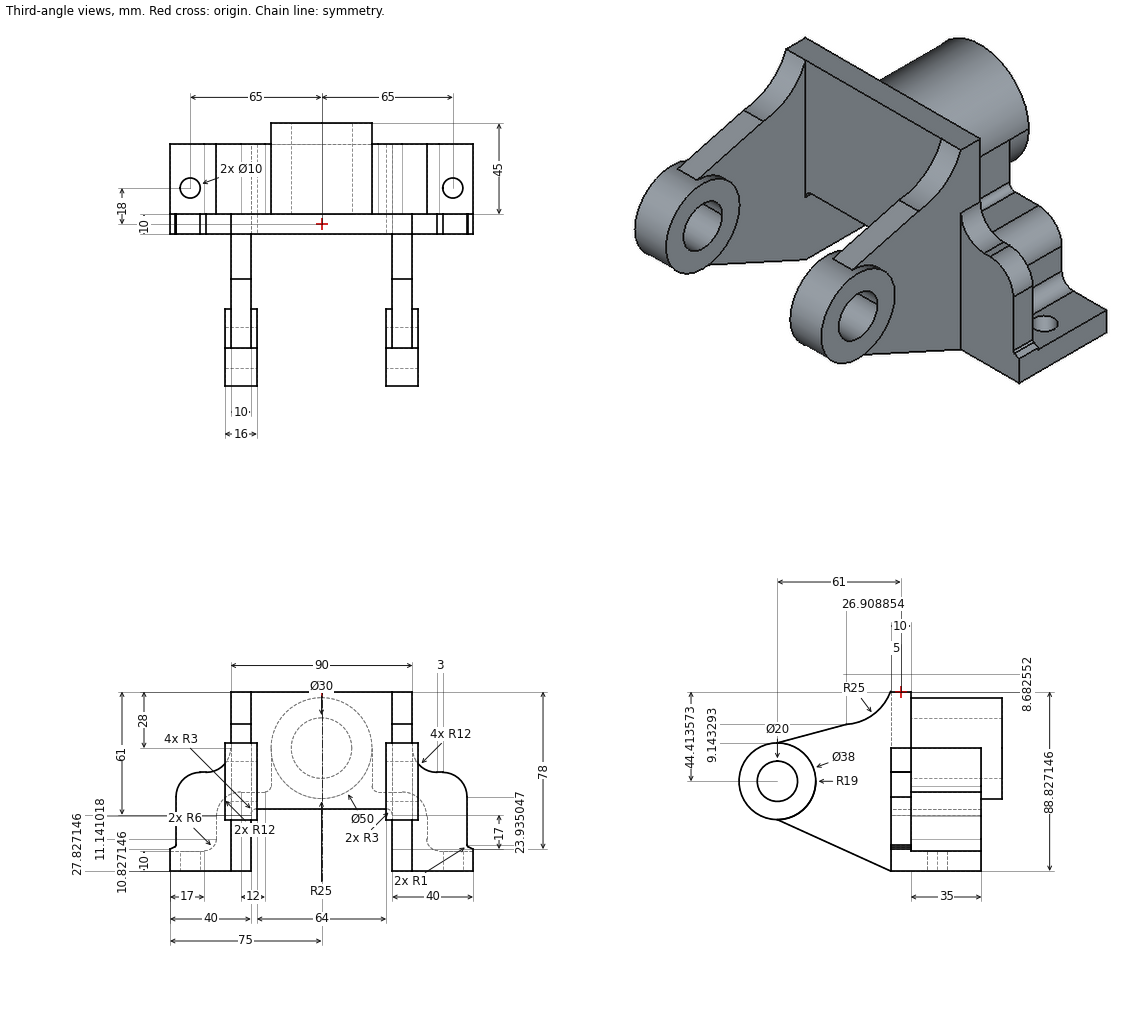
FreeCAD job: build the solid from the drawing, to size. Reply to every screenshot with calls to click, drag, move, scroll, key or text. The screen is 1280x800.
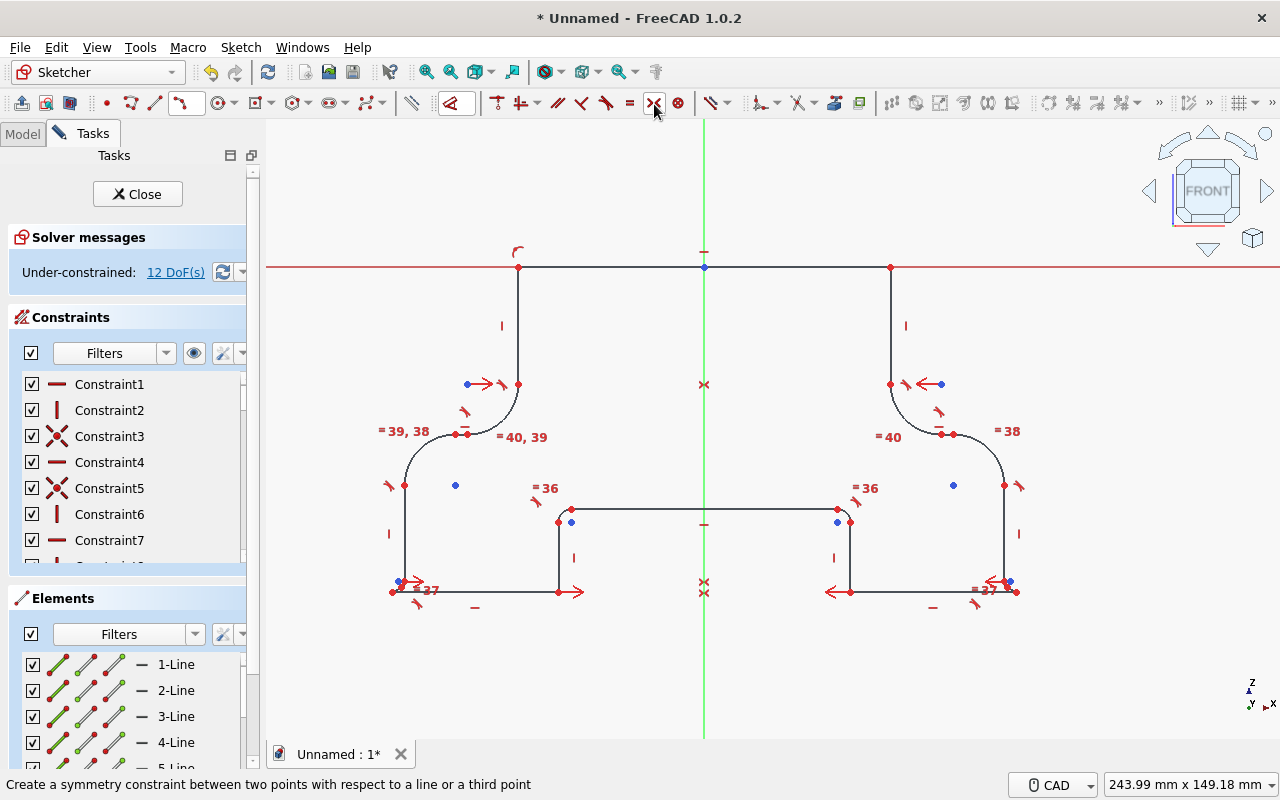
click(999, 462)
click(1028, 447)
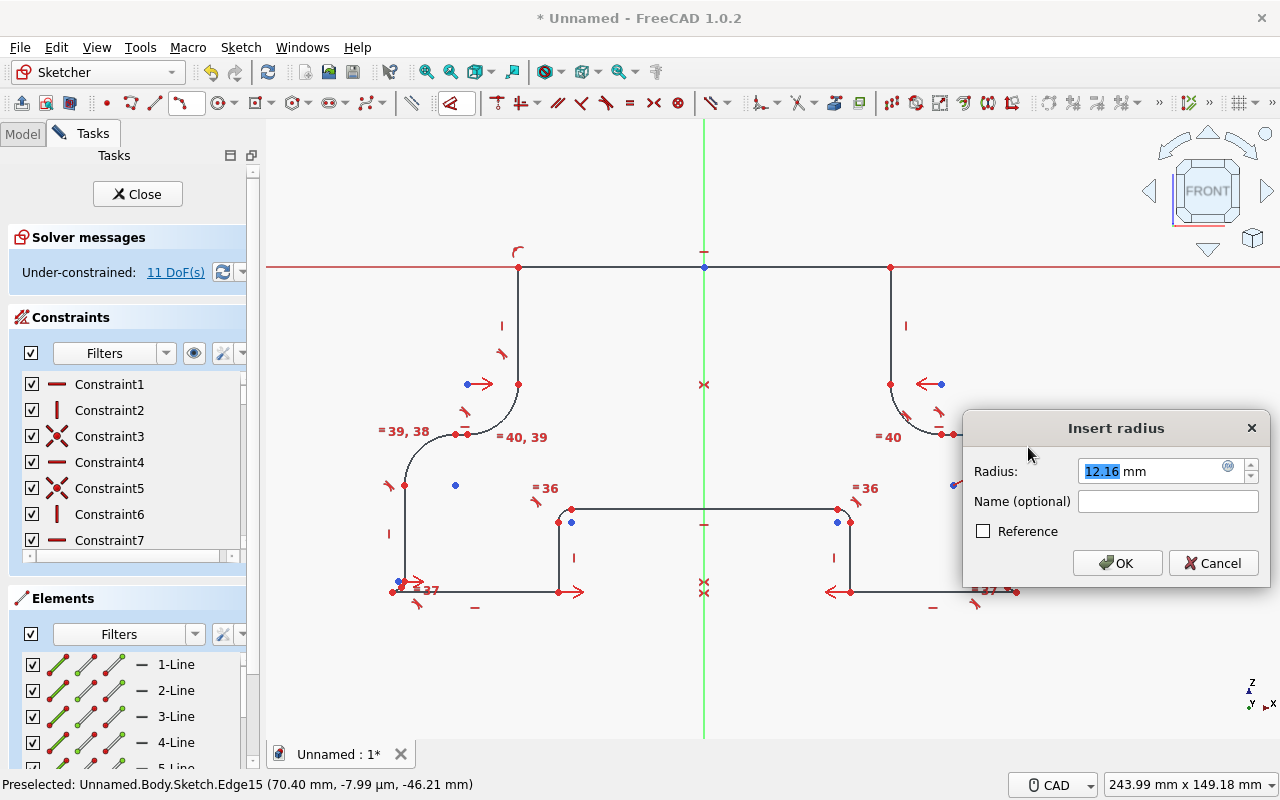
text(12)
key(Return)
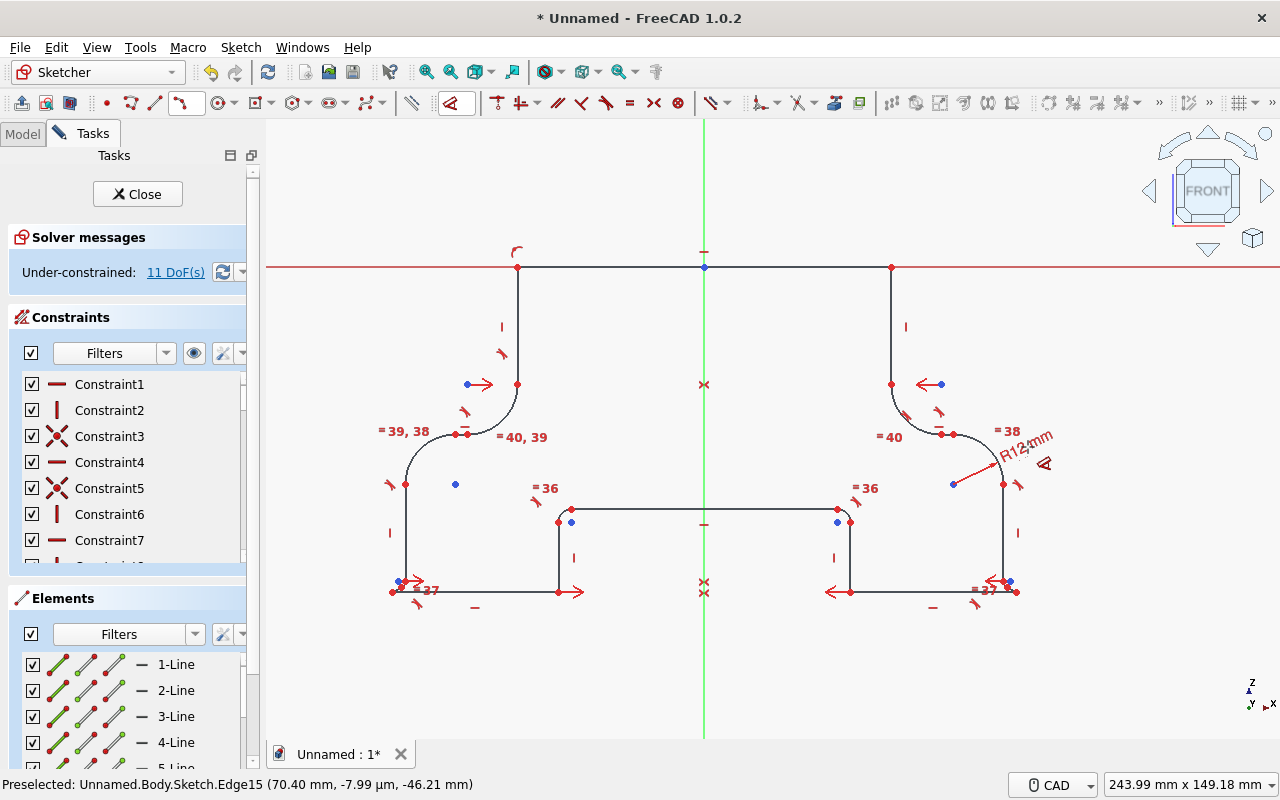
scroll(1004, 585, up, 12)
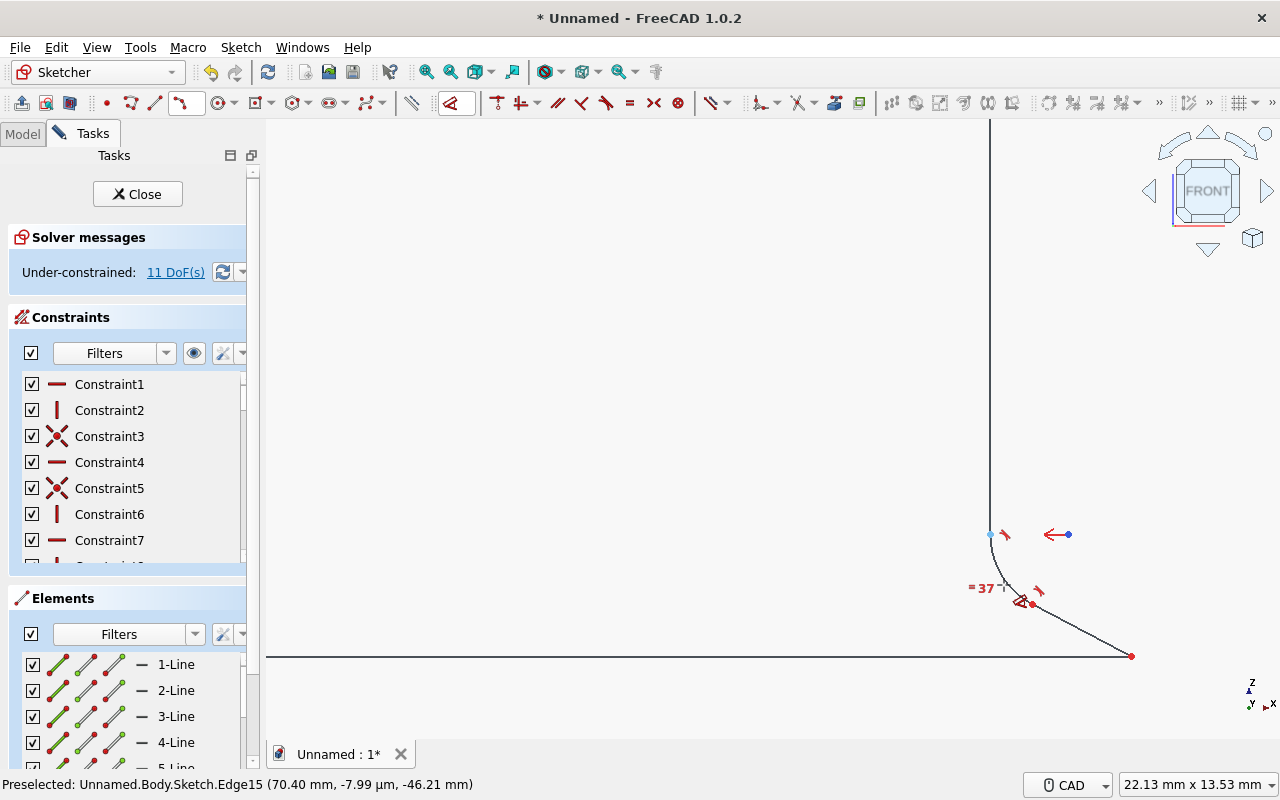
click(1002, 575)
click(975, 591)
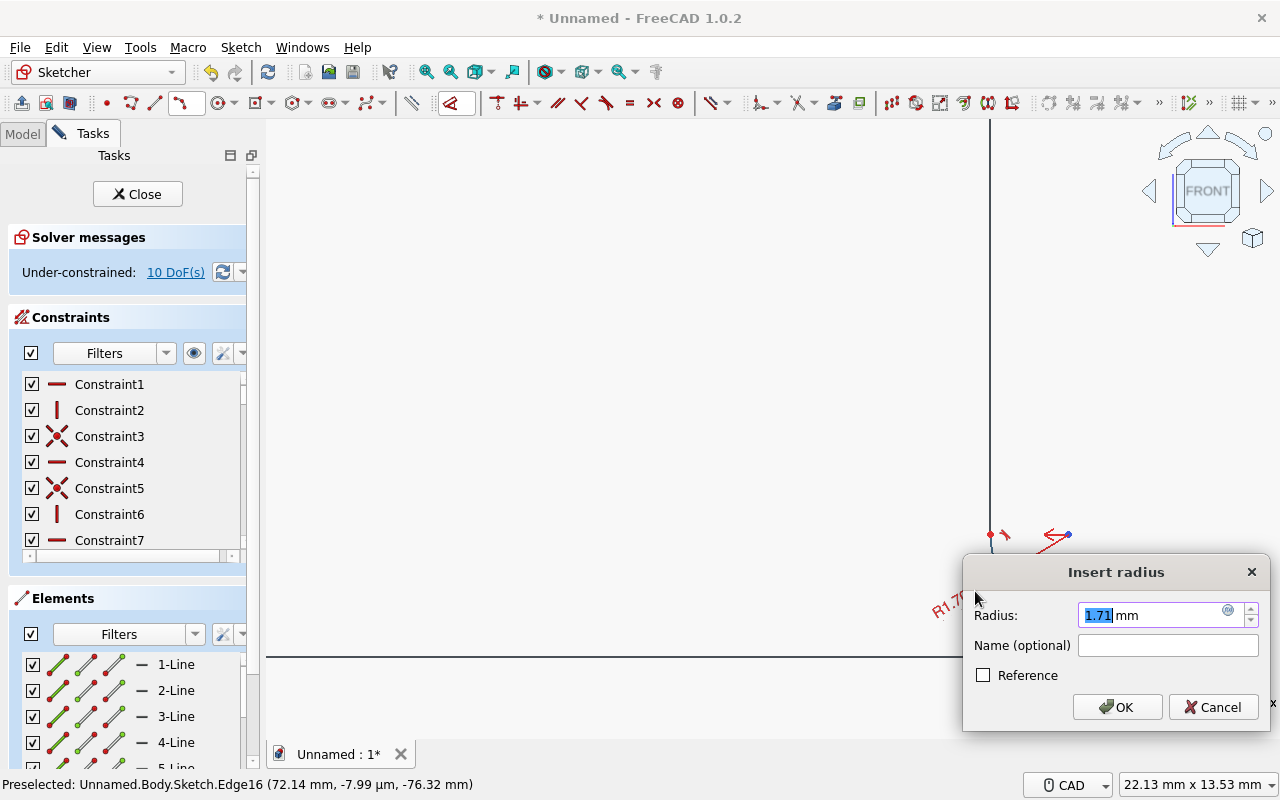
text(1)
key(Return)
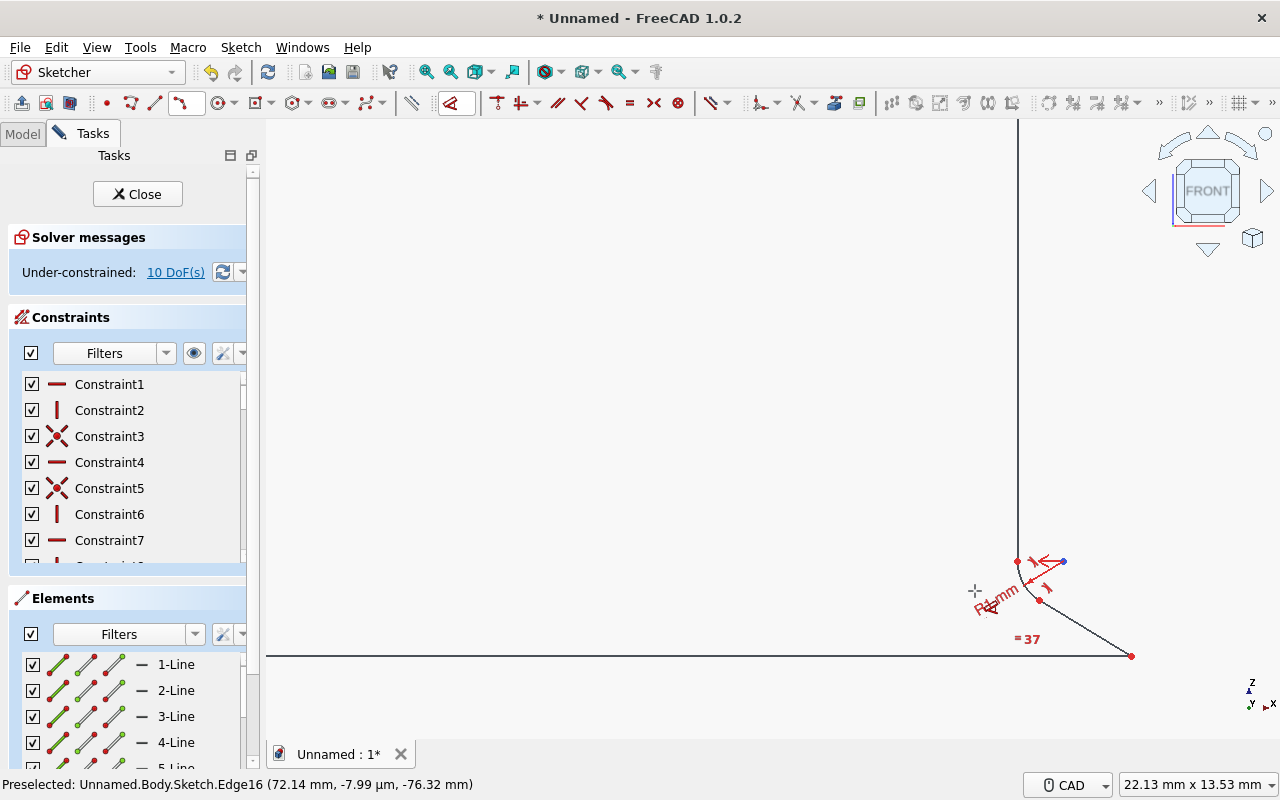
scroll(1005, 585, down, 12)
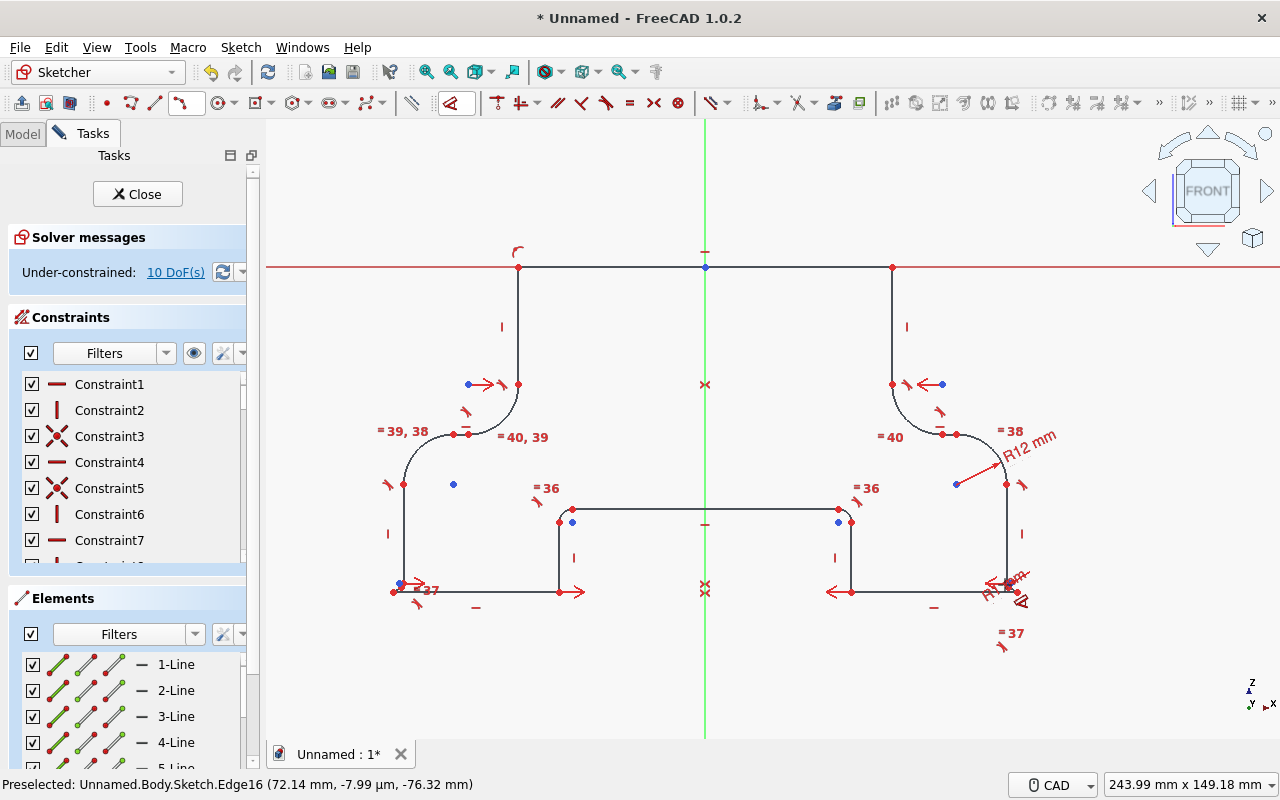
scroll(850, 516, up, 6)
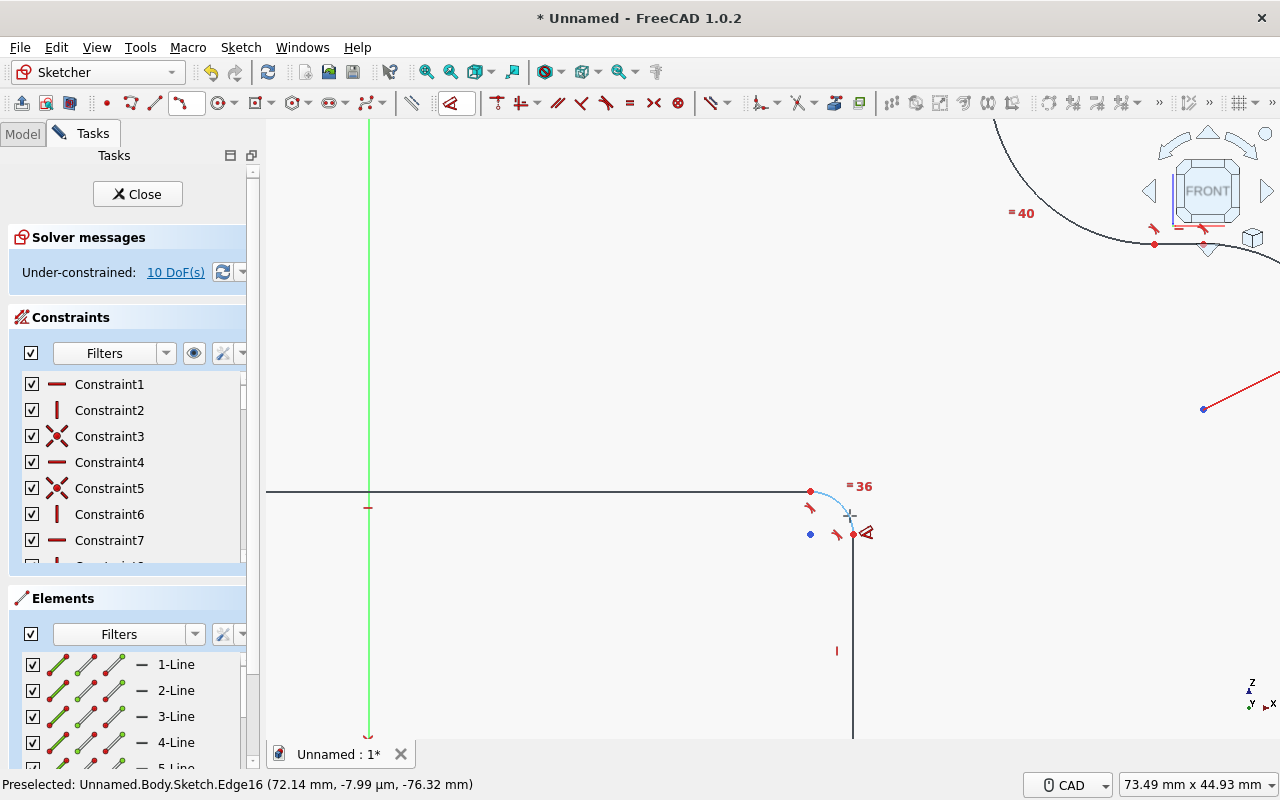
click(848, 515)
click(876, 500)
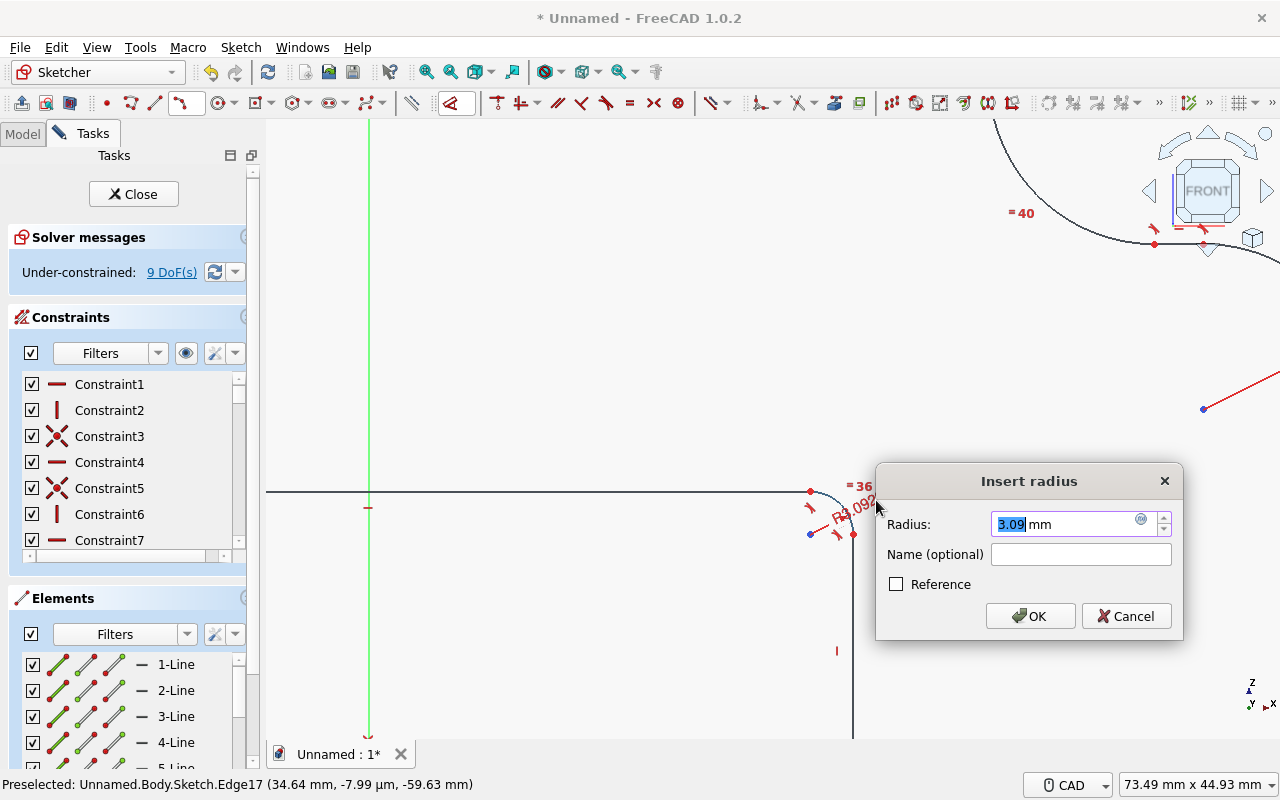
text(3)
key(Return)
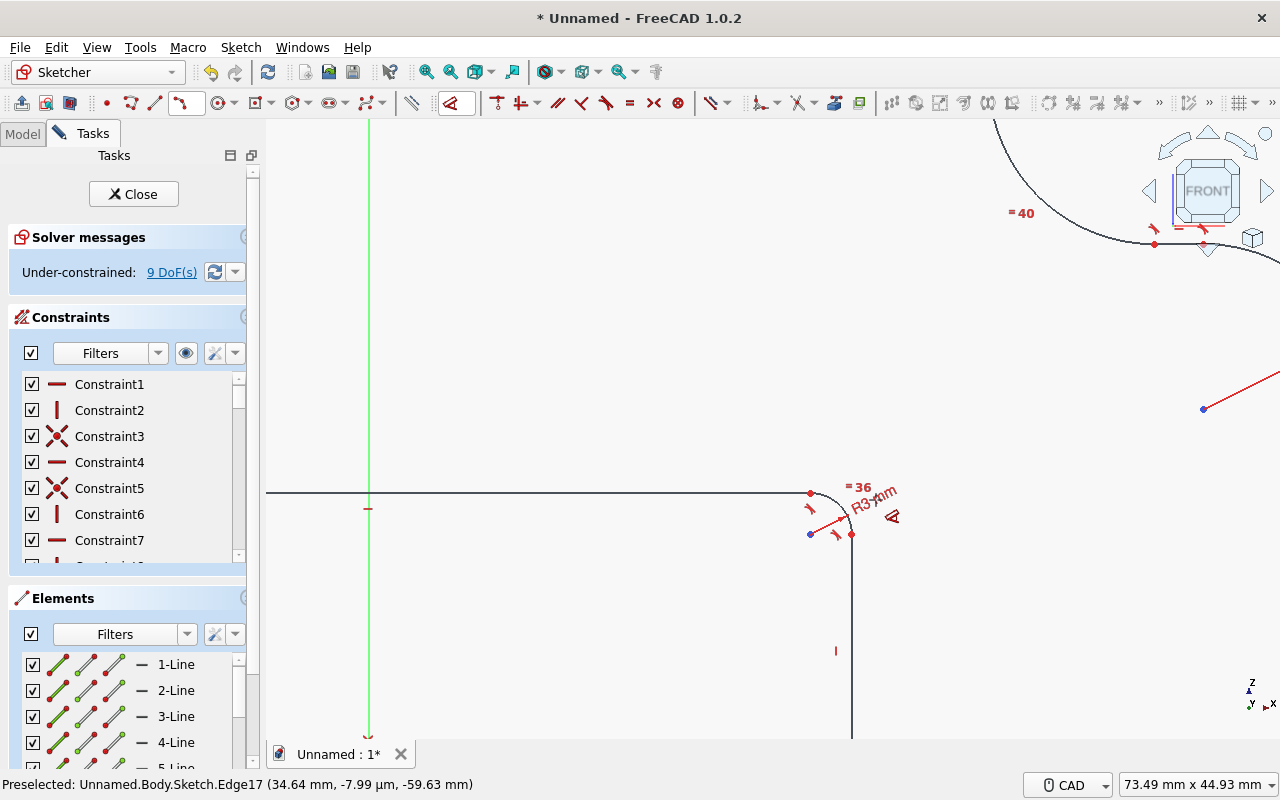
scroll(849, 516, down, 6)